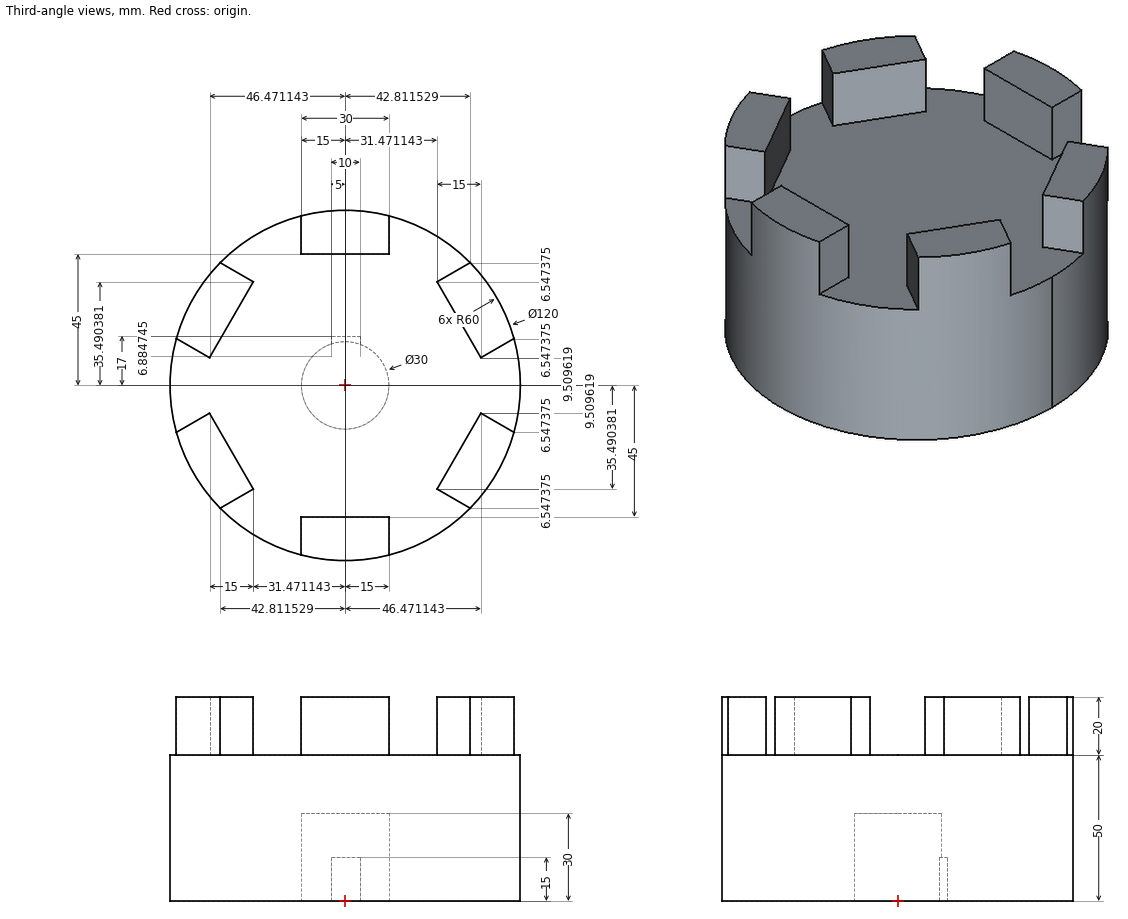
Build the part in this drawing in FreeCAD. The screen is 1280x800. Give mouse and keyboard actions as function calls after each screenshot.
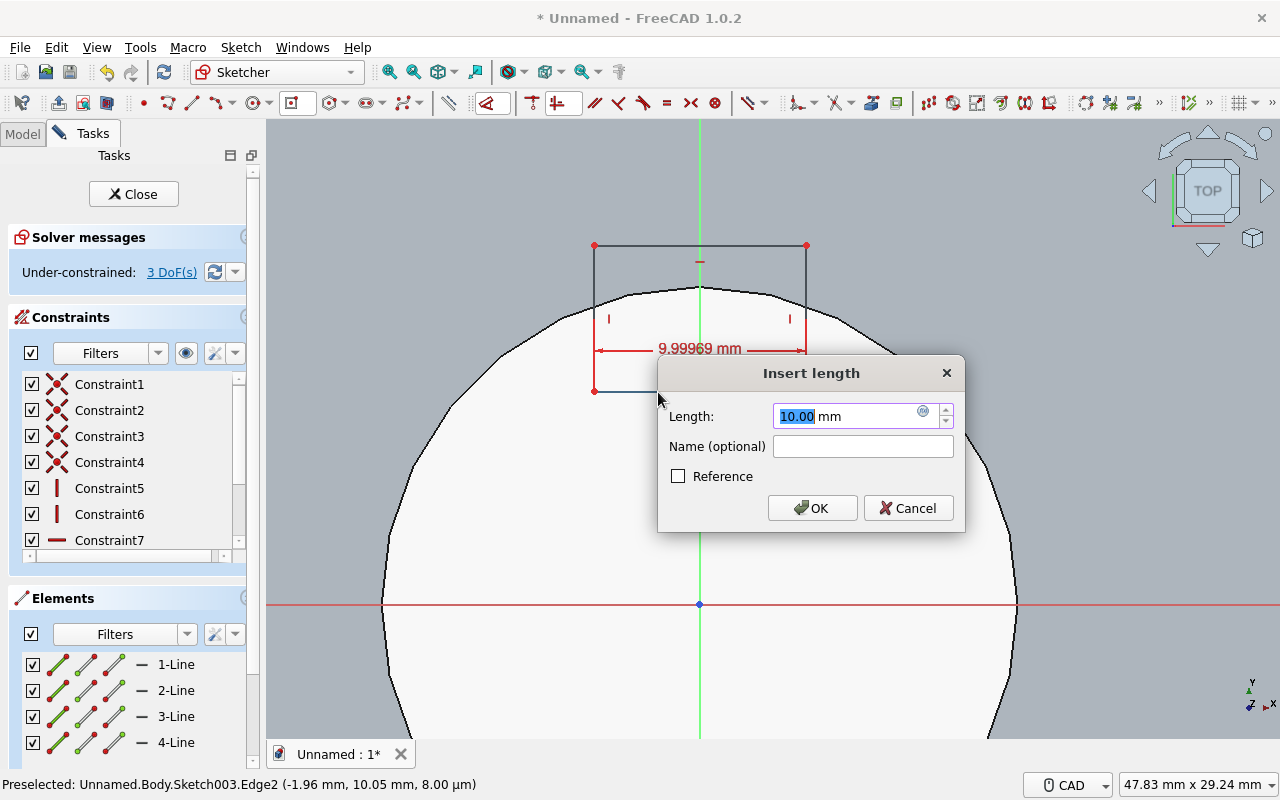
text(10)
key(Return)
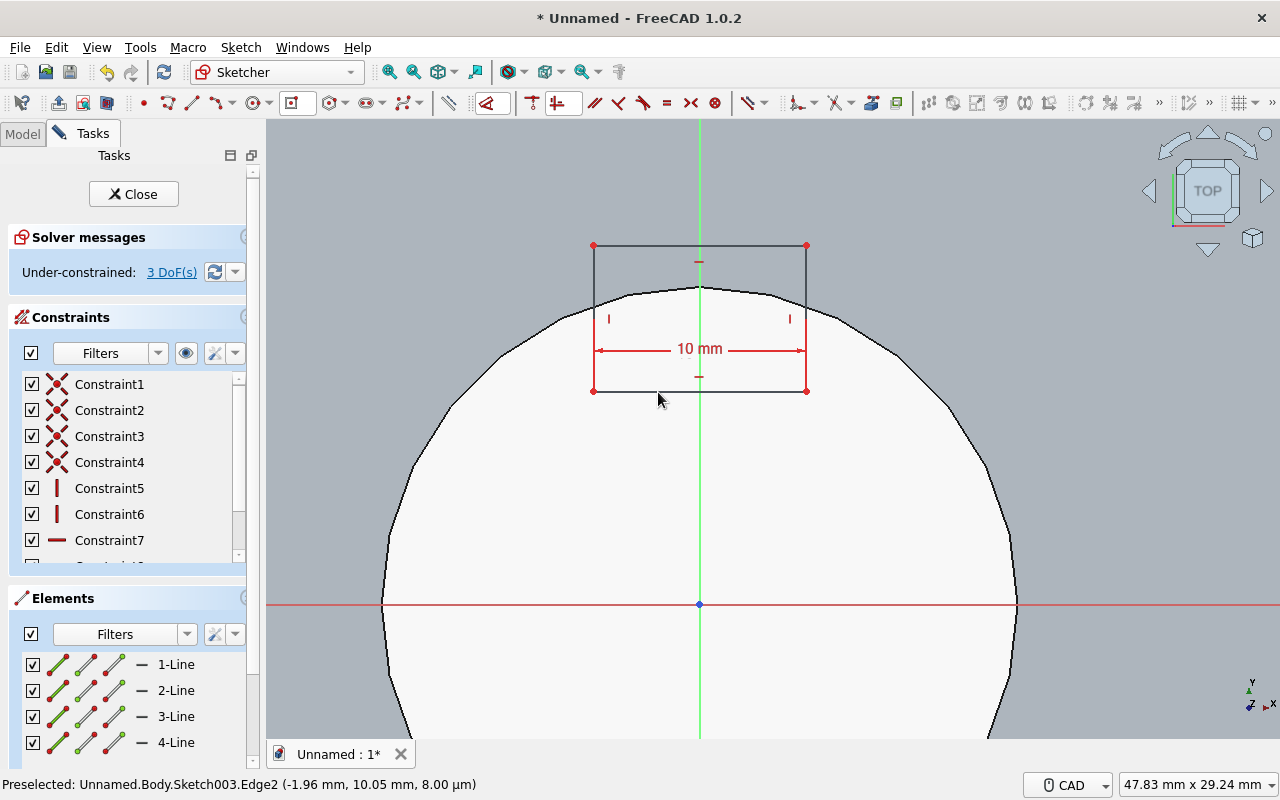
click(594, 246)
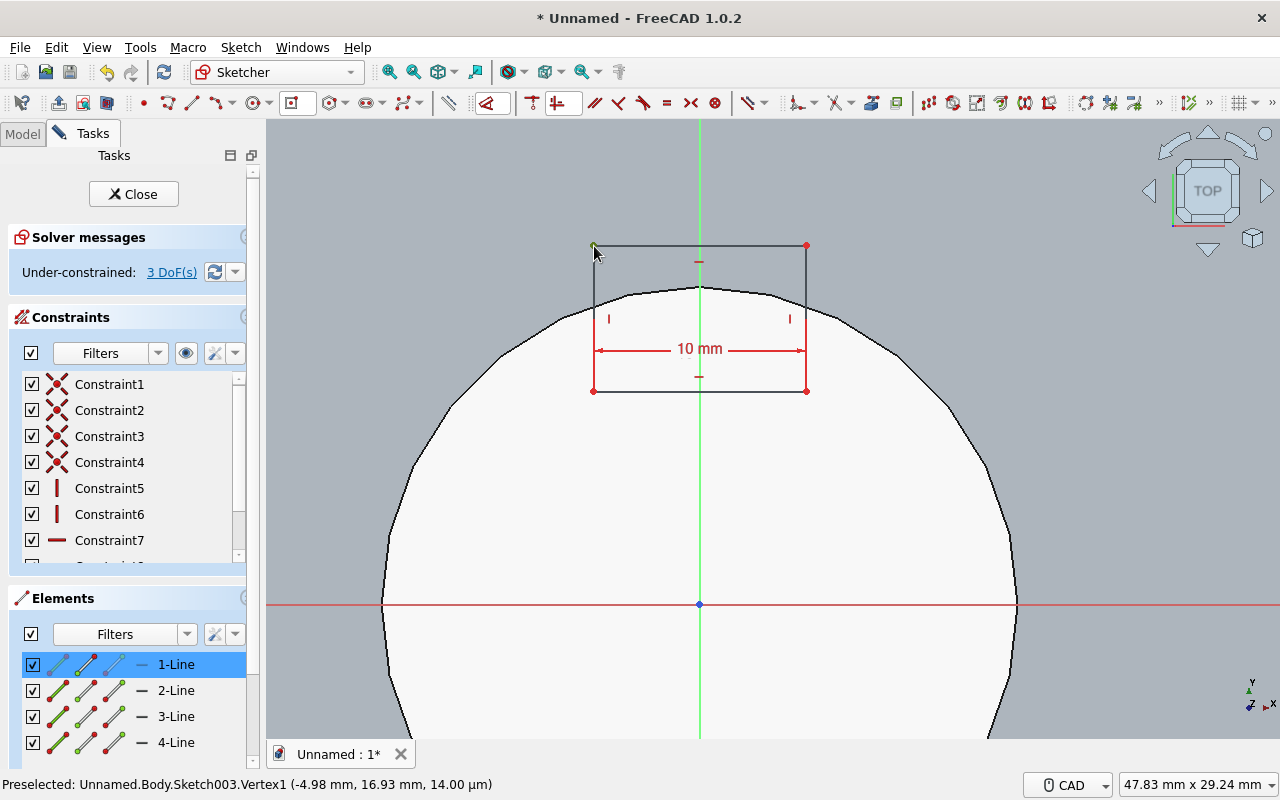
key(l)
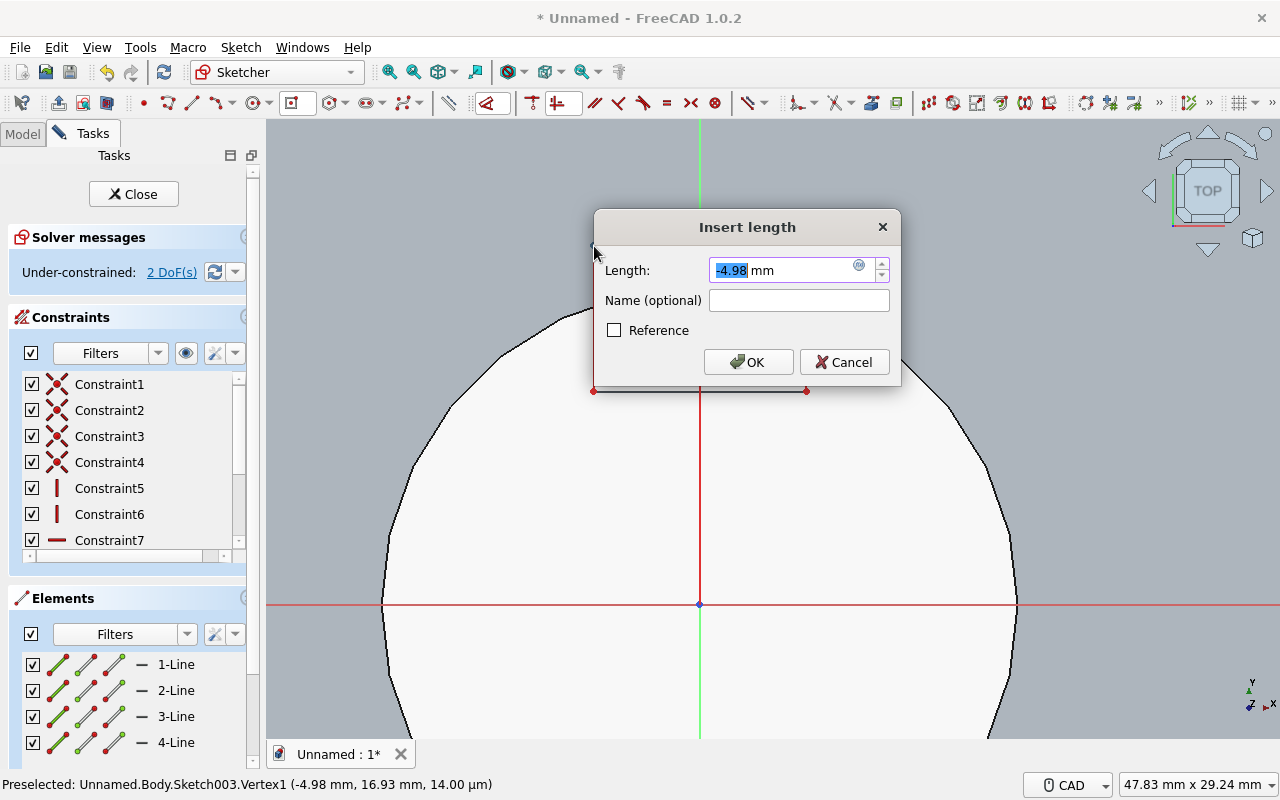
text(-5)
key(Return)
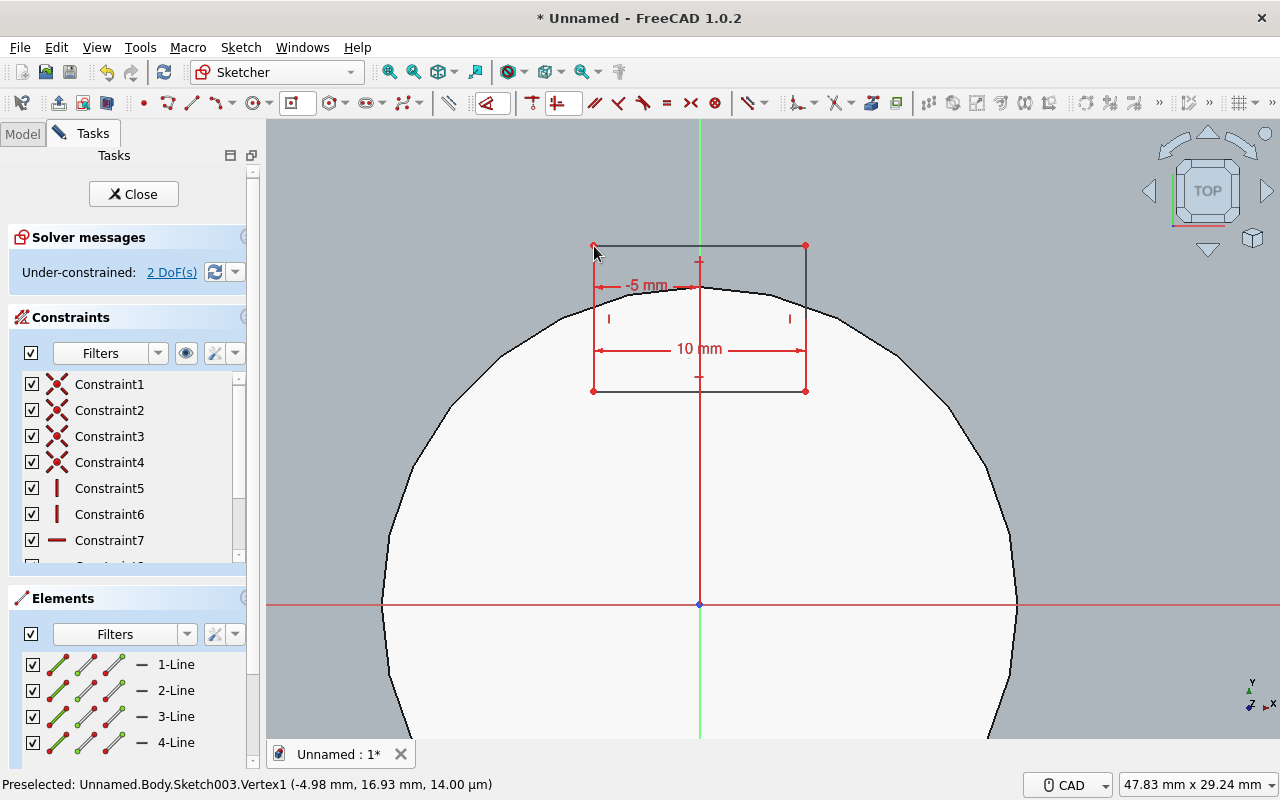
click(594, 246)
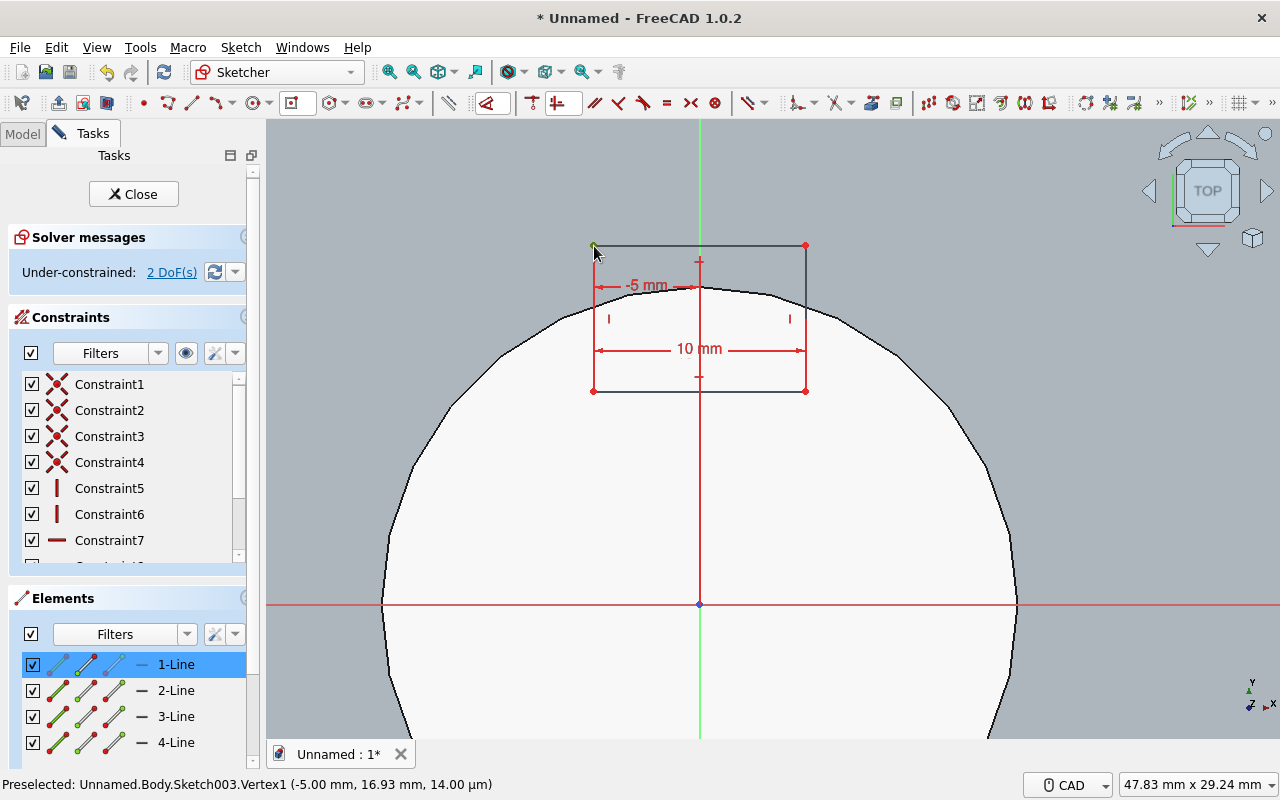
key(i)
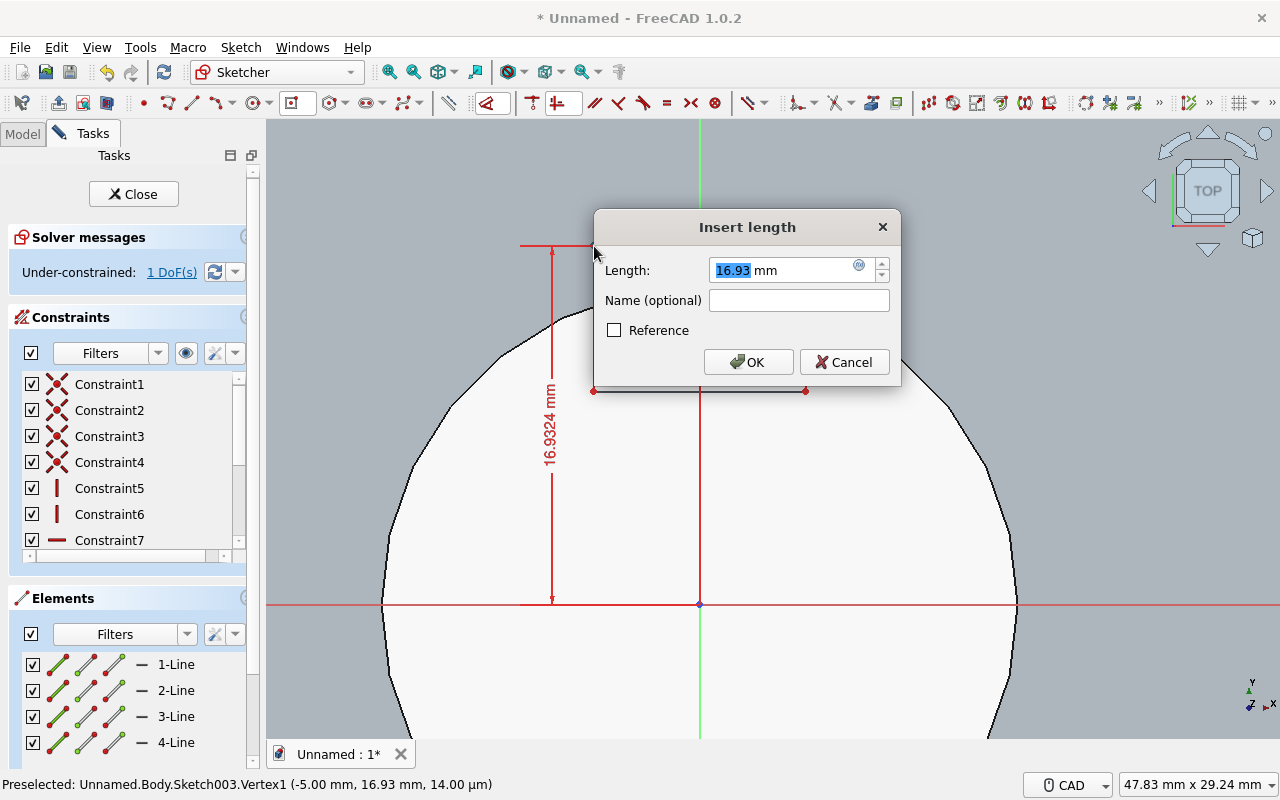
text(17)
key(Return)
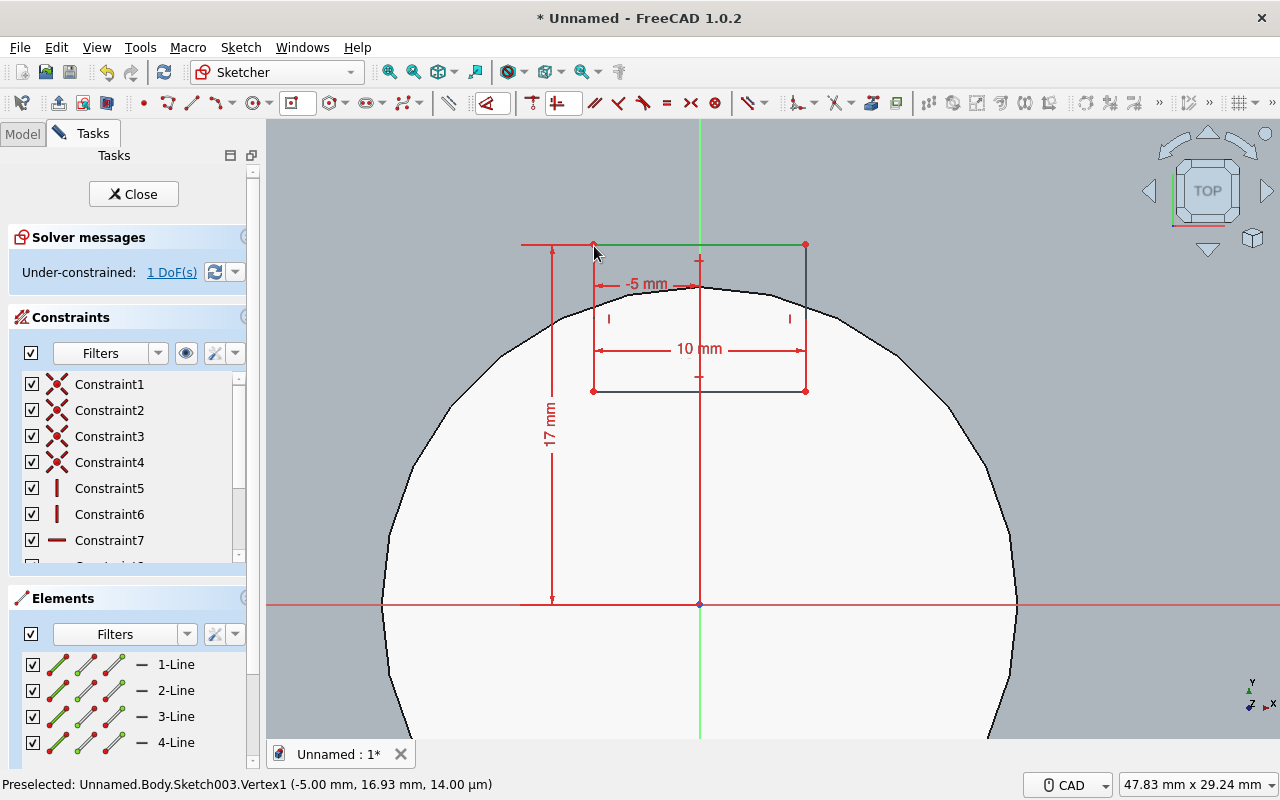
click(594, 289)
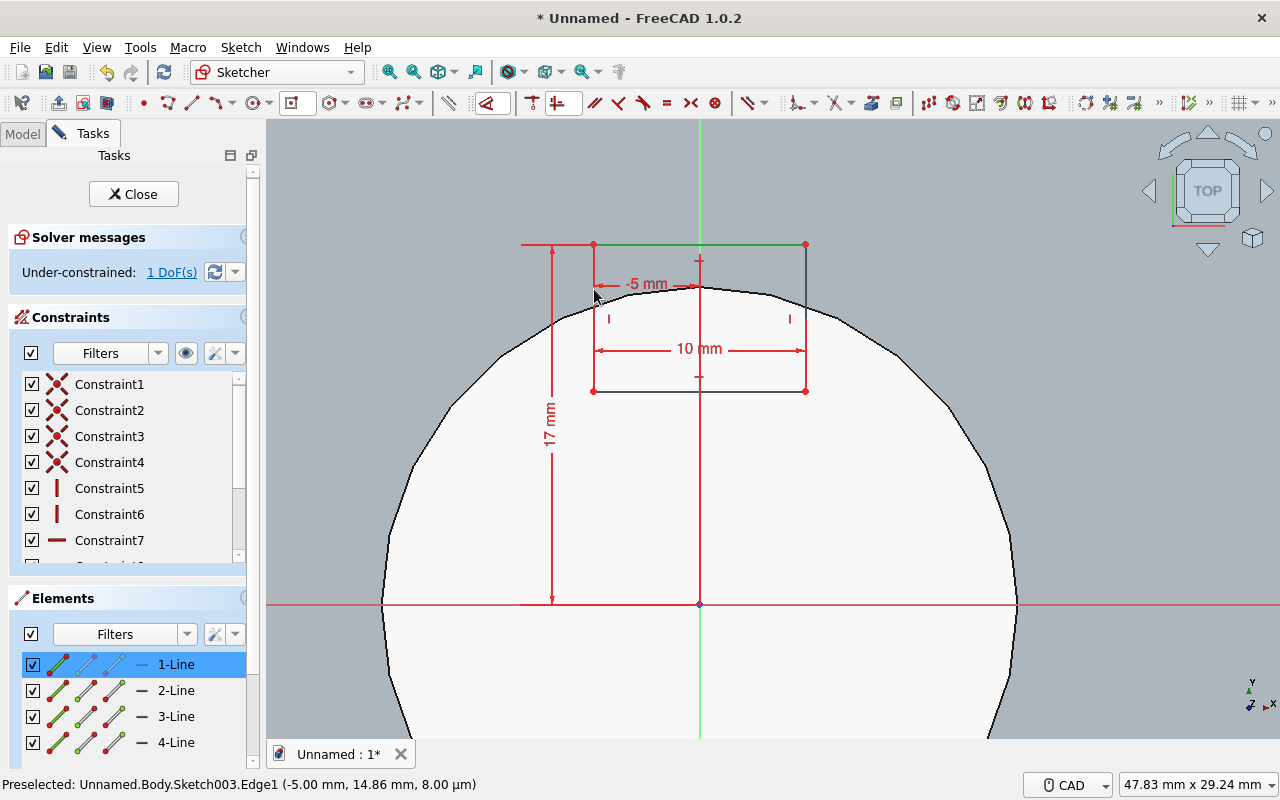
key(i)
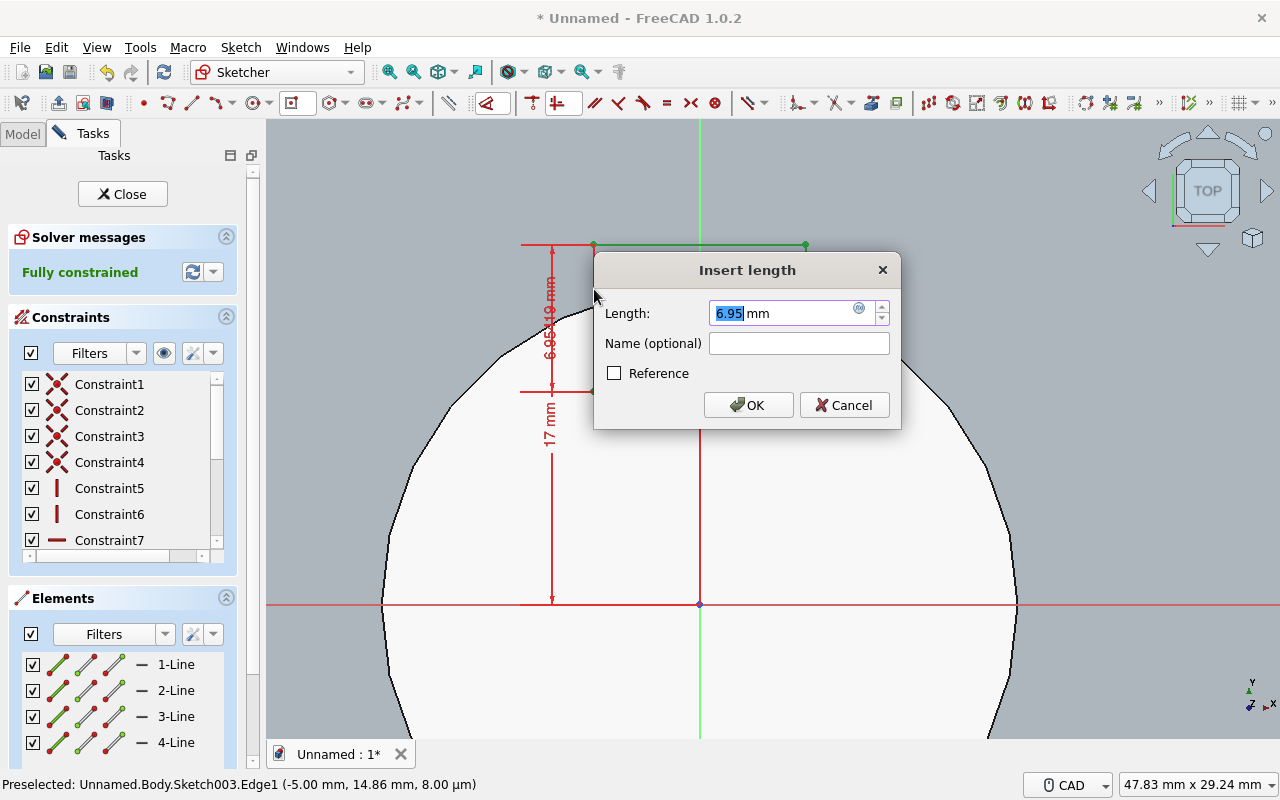
text(6.884745)
key(Return)